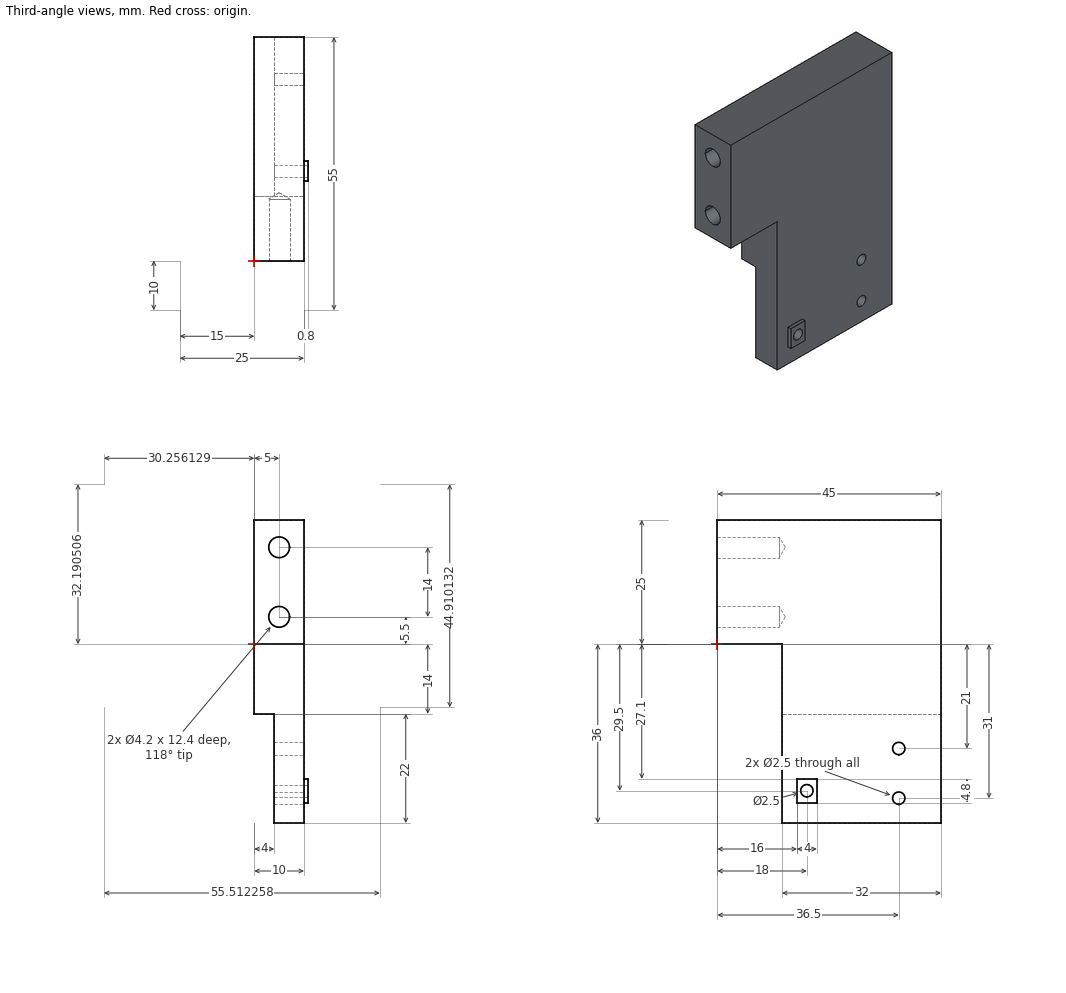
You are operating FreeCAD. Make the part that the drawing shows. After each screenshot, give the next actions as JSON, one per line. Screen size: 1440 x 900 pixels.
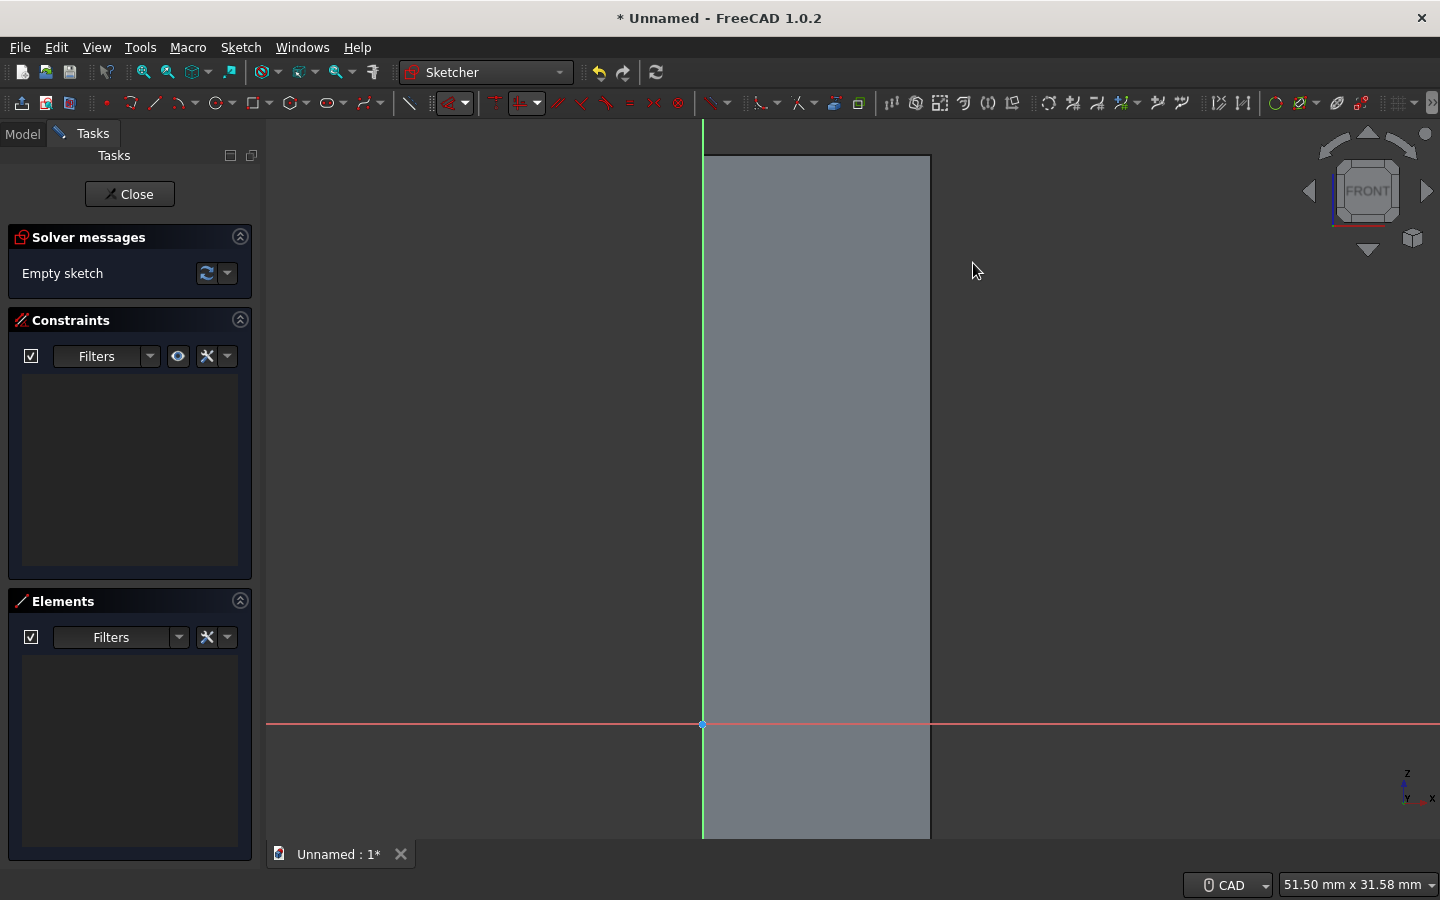
{"action": "left_click", "coordinate": [216, 104]}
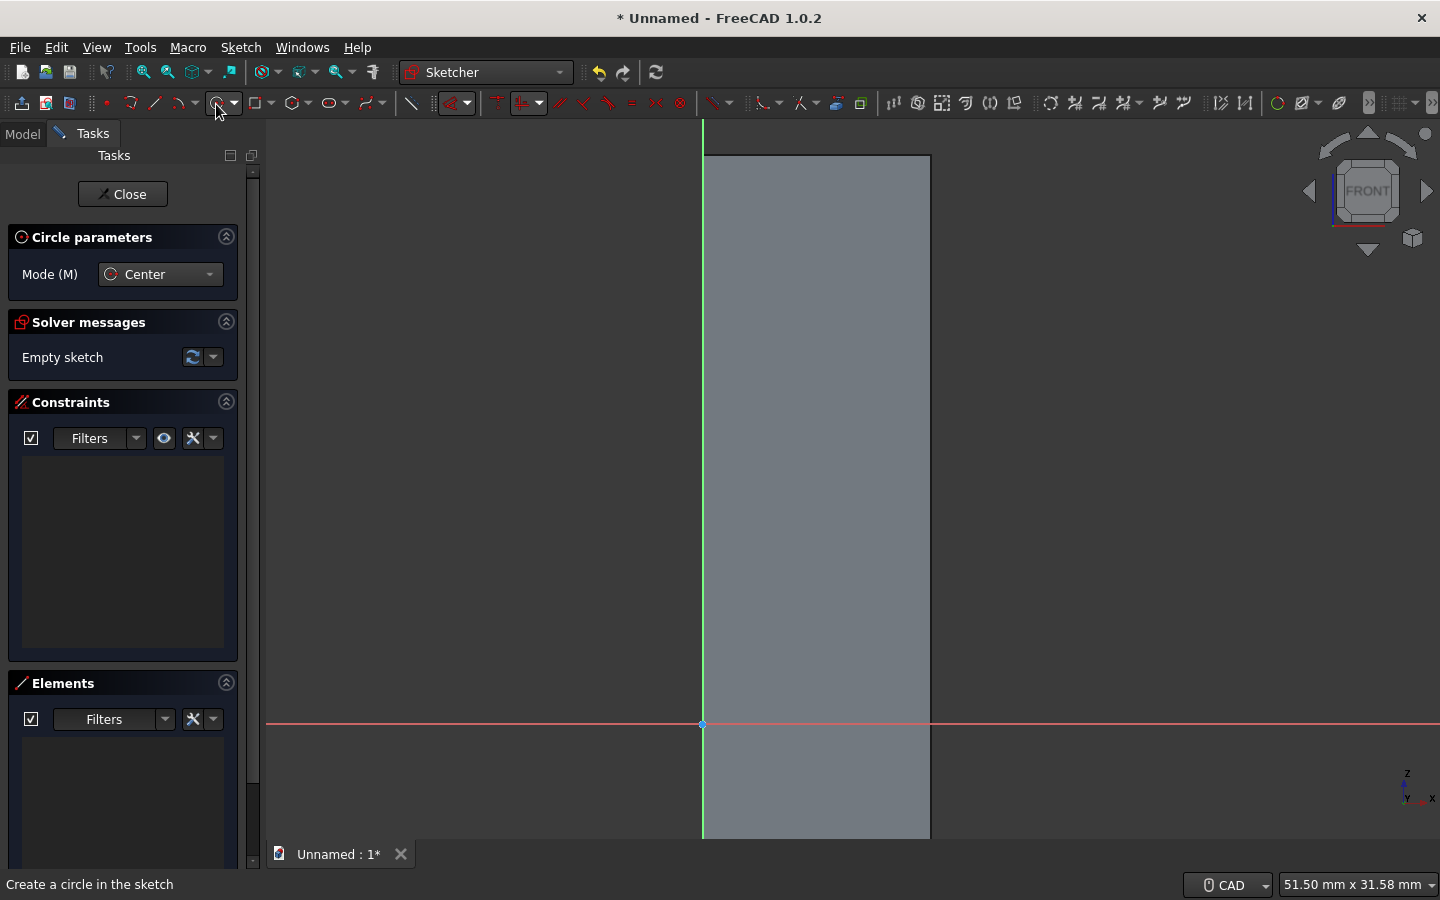
{"action": "left_click", "coordinate": [817, 599]}
{"action": "mouse_move", "coordinate": [851, 565]}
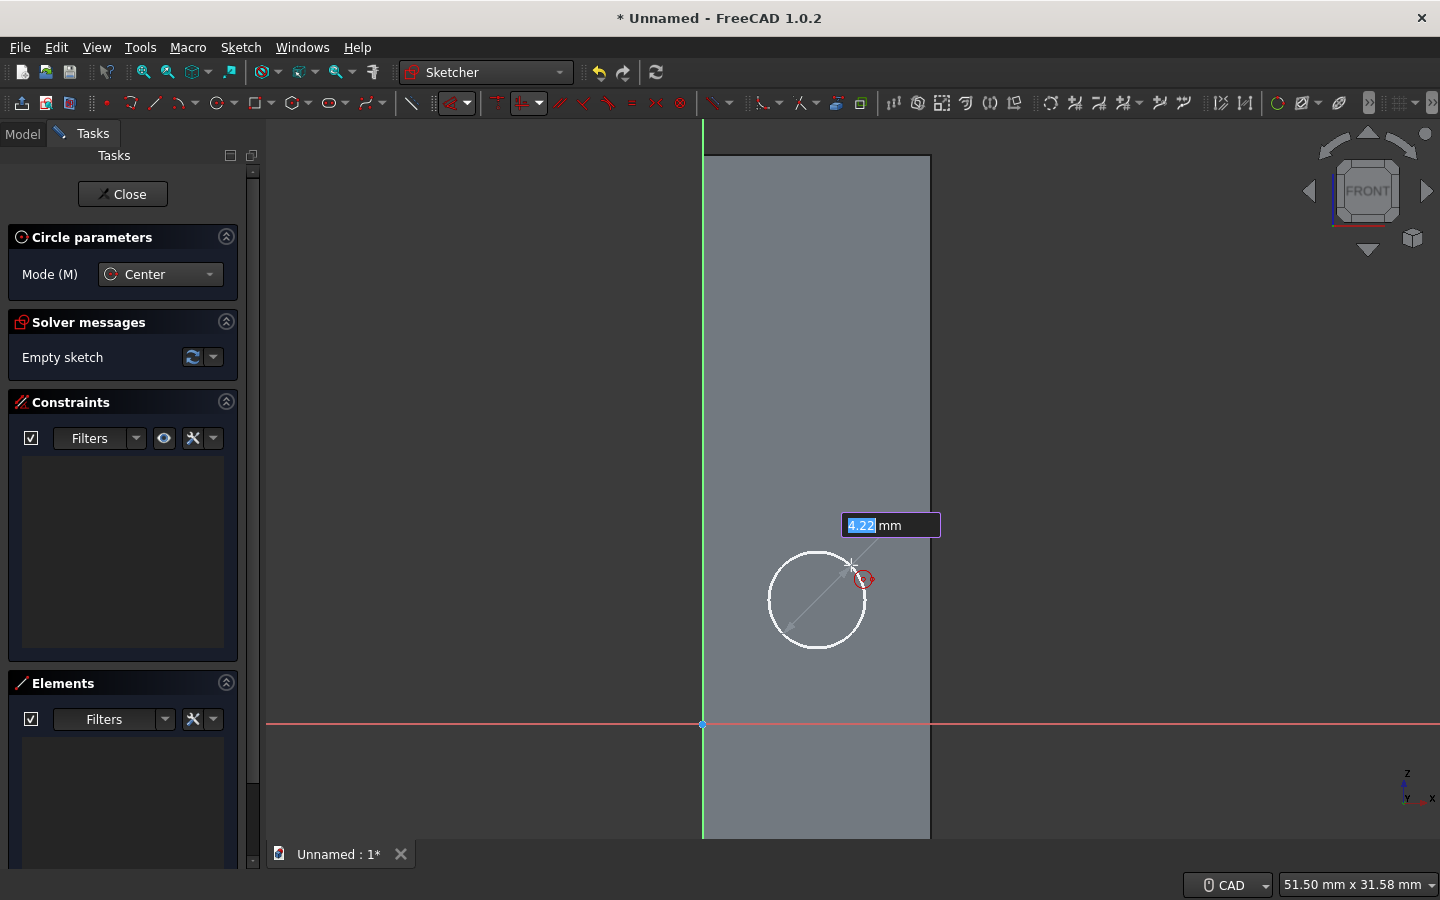
{"action": "type", "text": "4.2"}
{"action": "key", "text": "Return"}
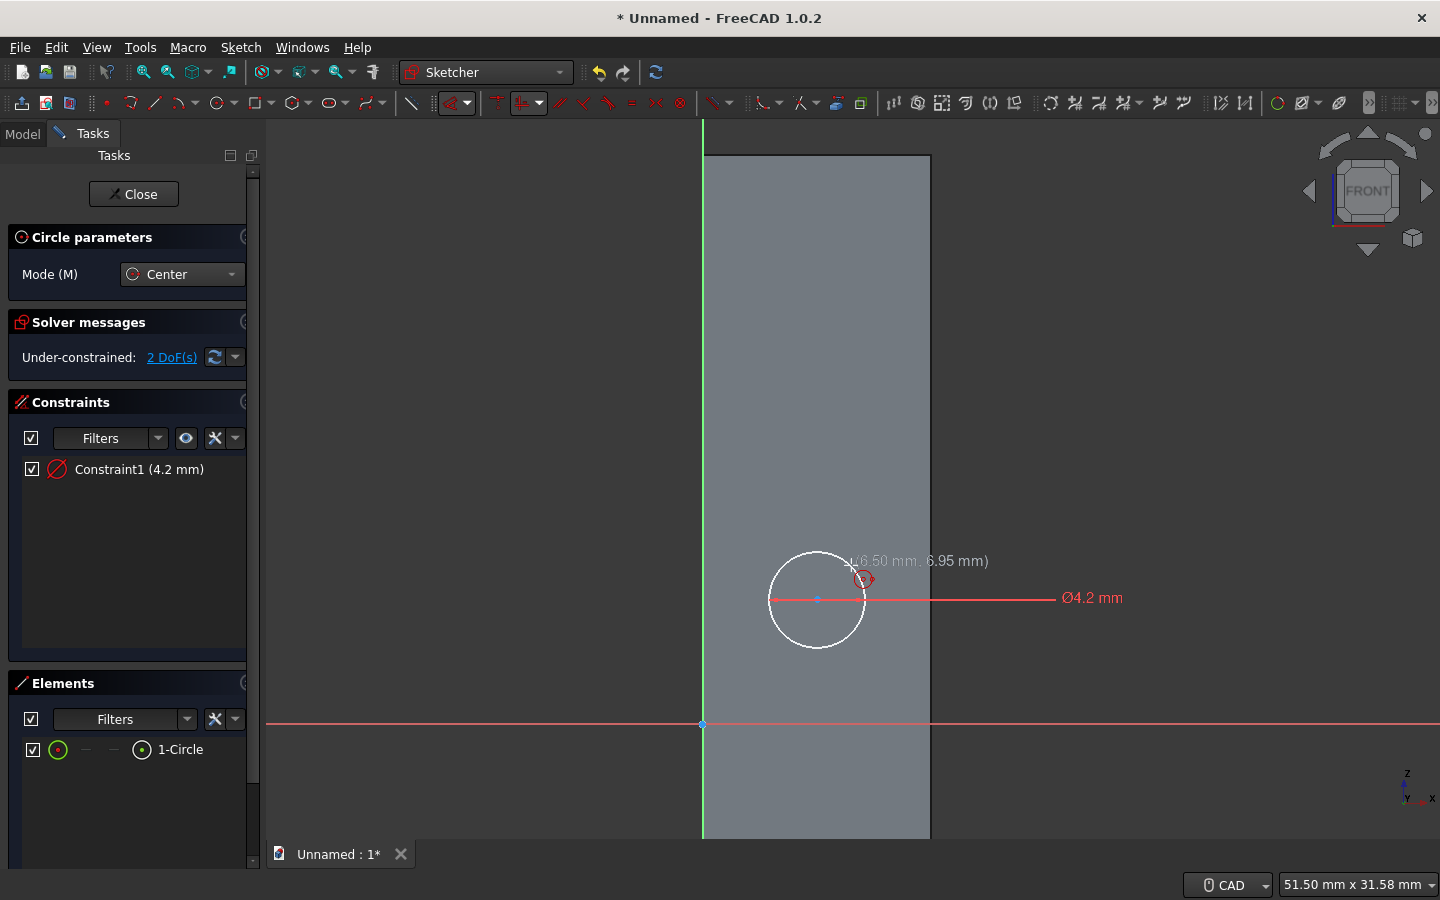
{"action": "left_click", "coordinate": [817, 280]}
{"action": "mouse_move", "coordinate": [851, 246]}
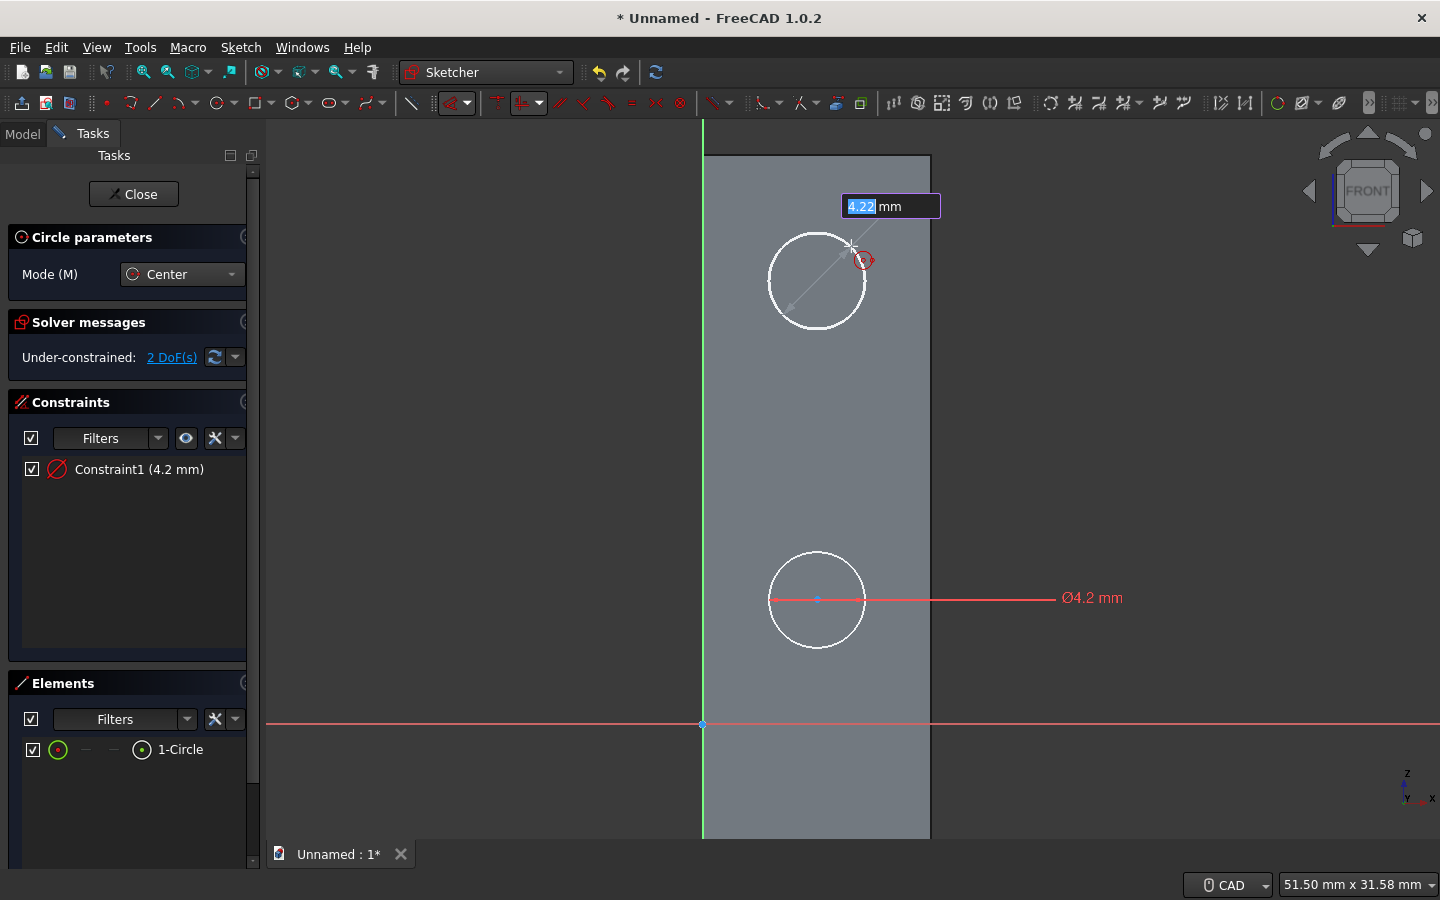
{"action": "type", "text": "4.2"}
{"action": "key", "text": "Return"}
{"action": "key", "text": "Escape"}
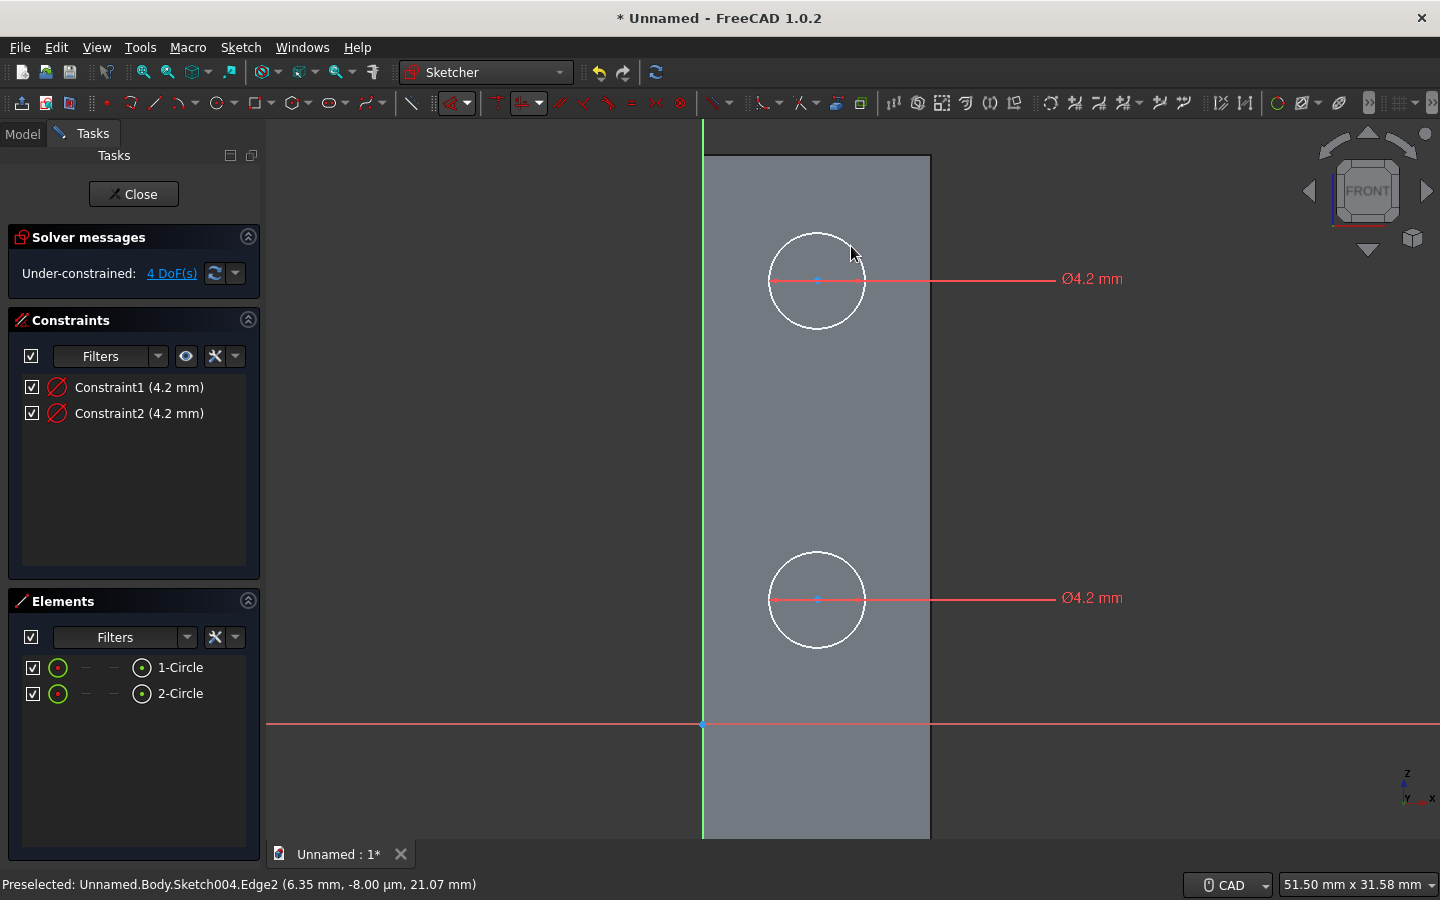
{"action": "left_click", "coordinate": [817, 600]}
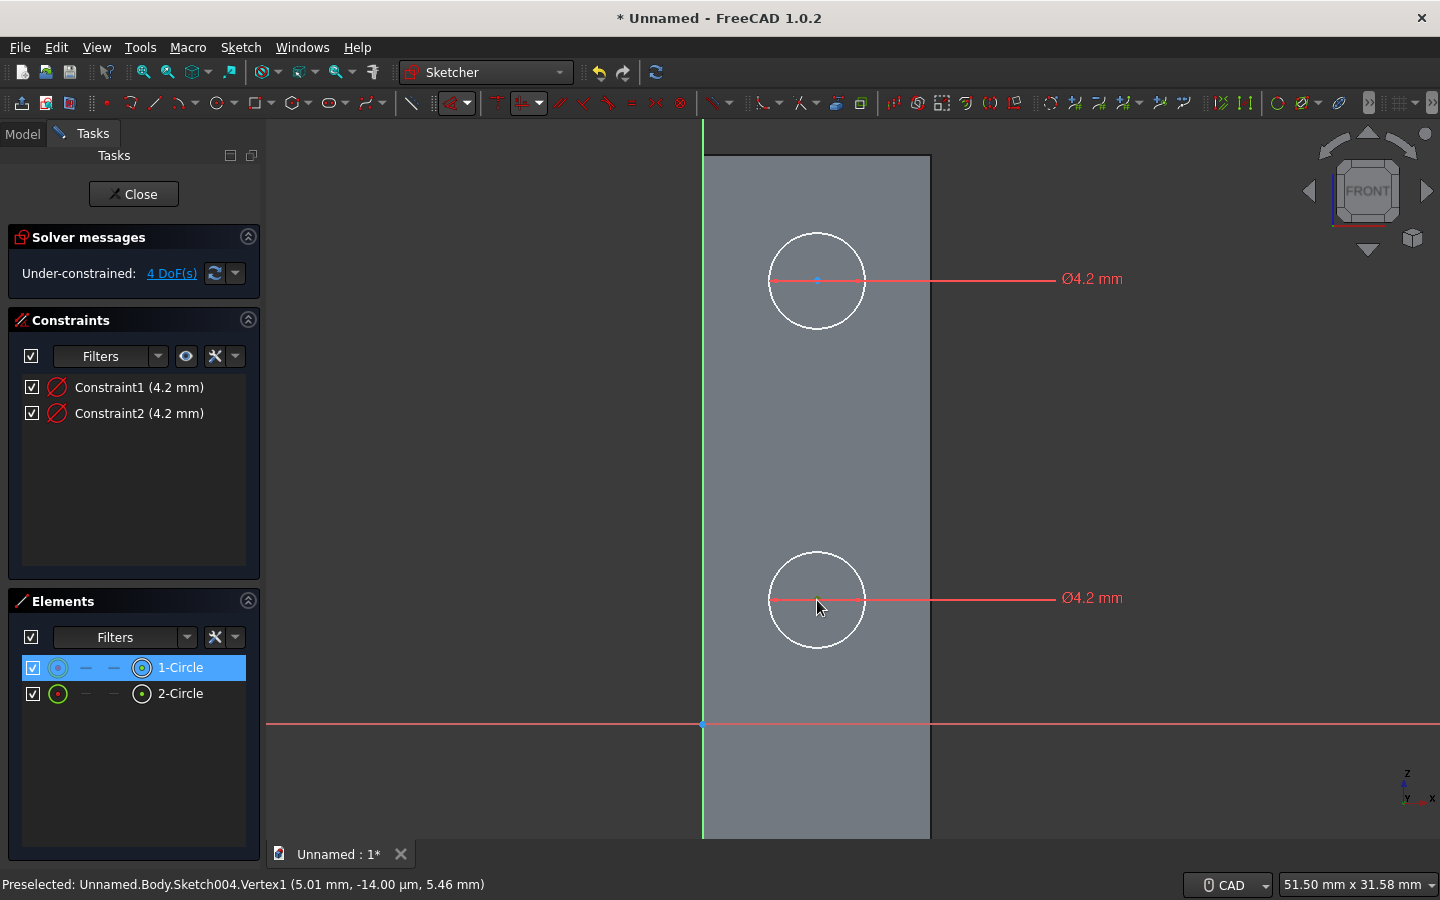
{"action": "left_click", "coordinate": [817, 281]}